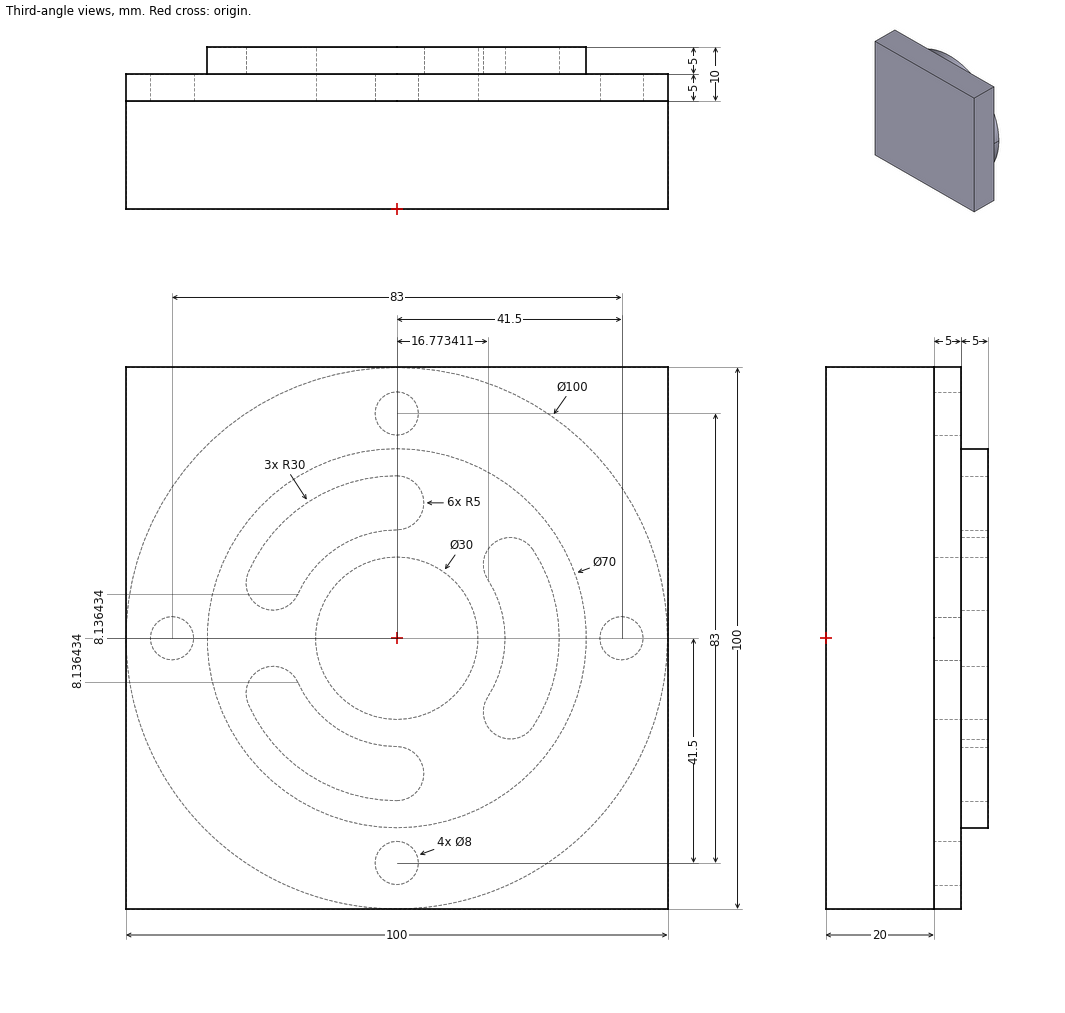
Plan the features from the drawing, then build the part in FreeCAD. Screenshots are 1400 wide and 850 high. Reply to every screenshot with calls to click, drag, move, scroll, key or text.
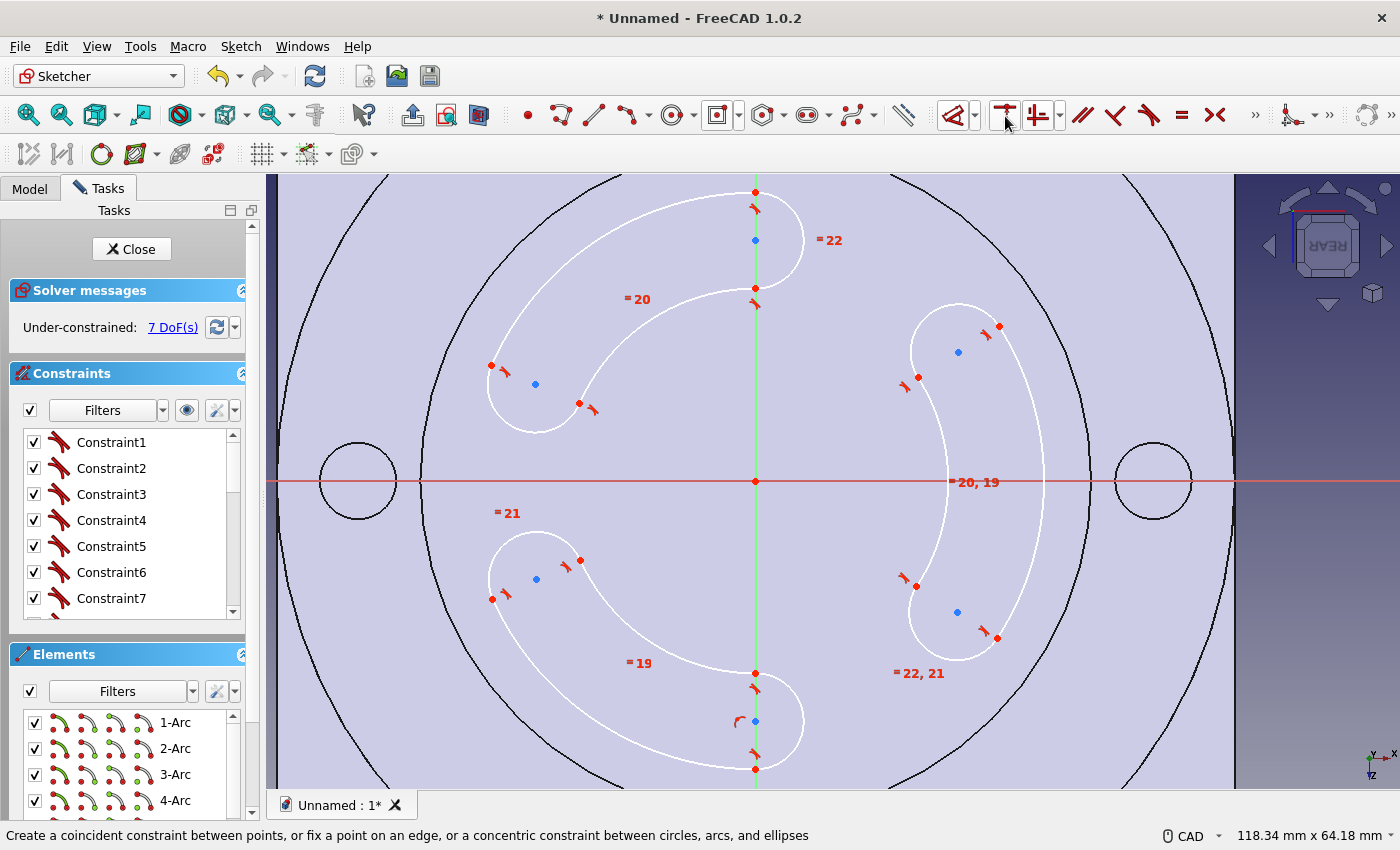
click(756, 241)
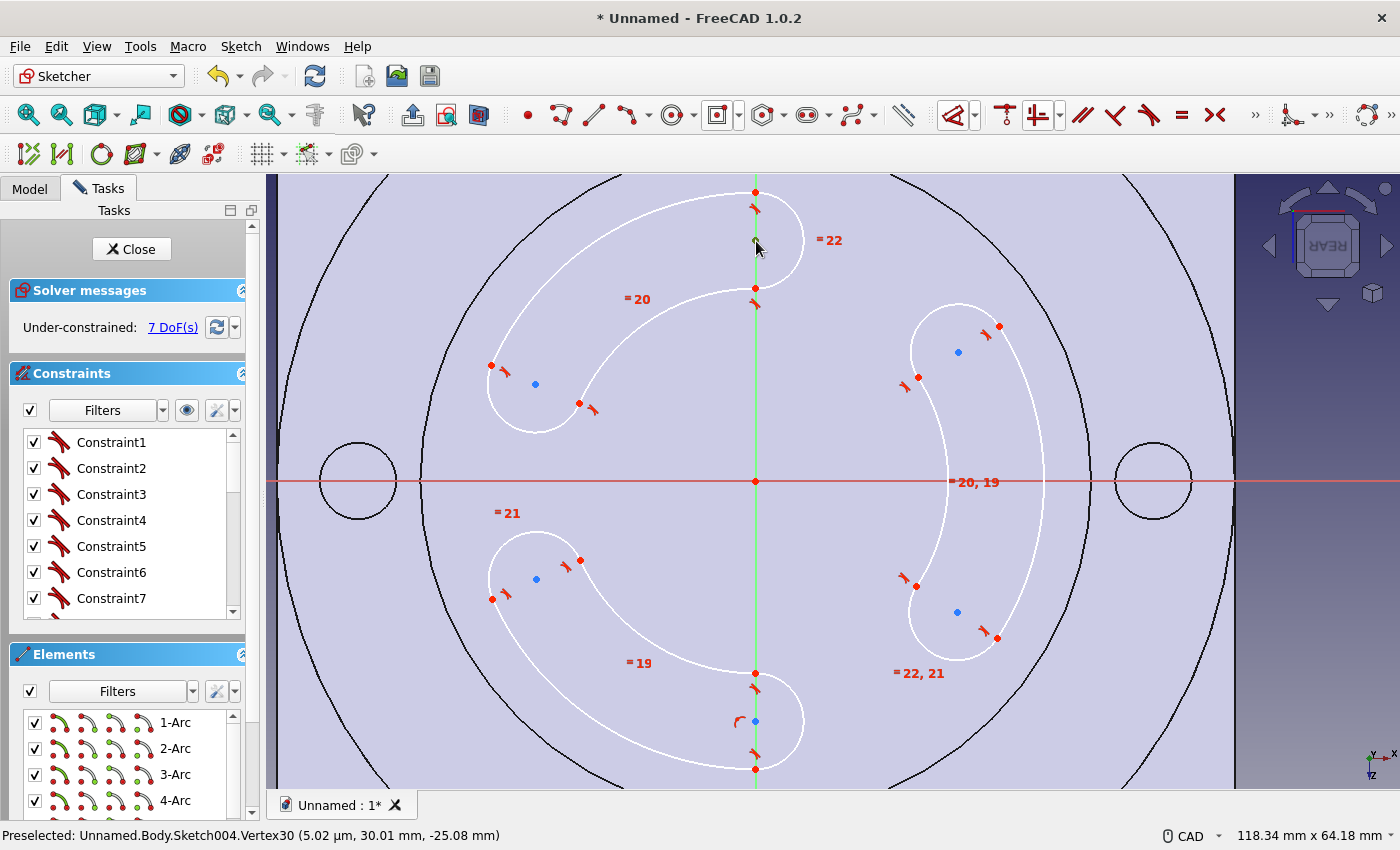
click(756, 641)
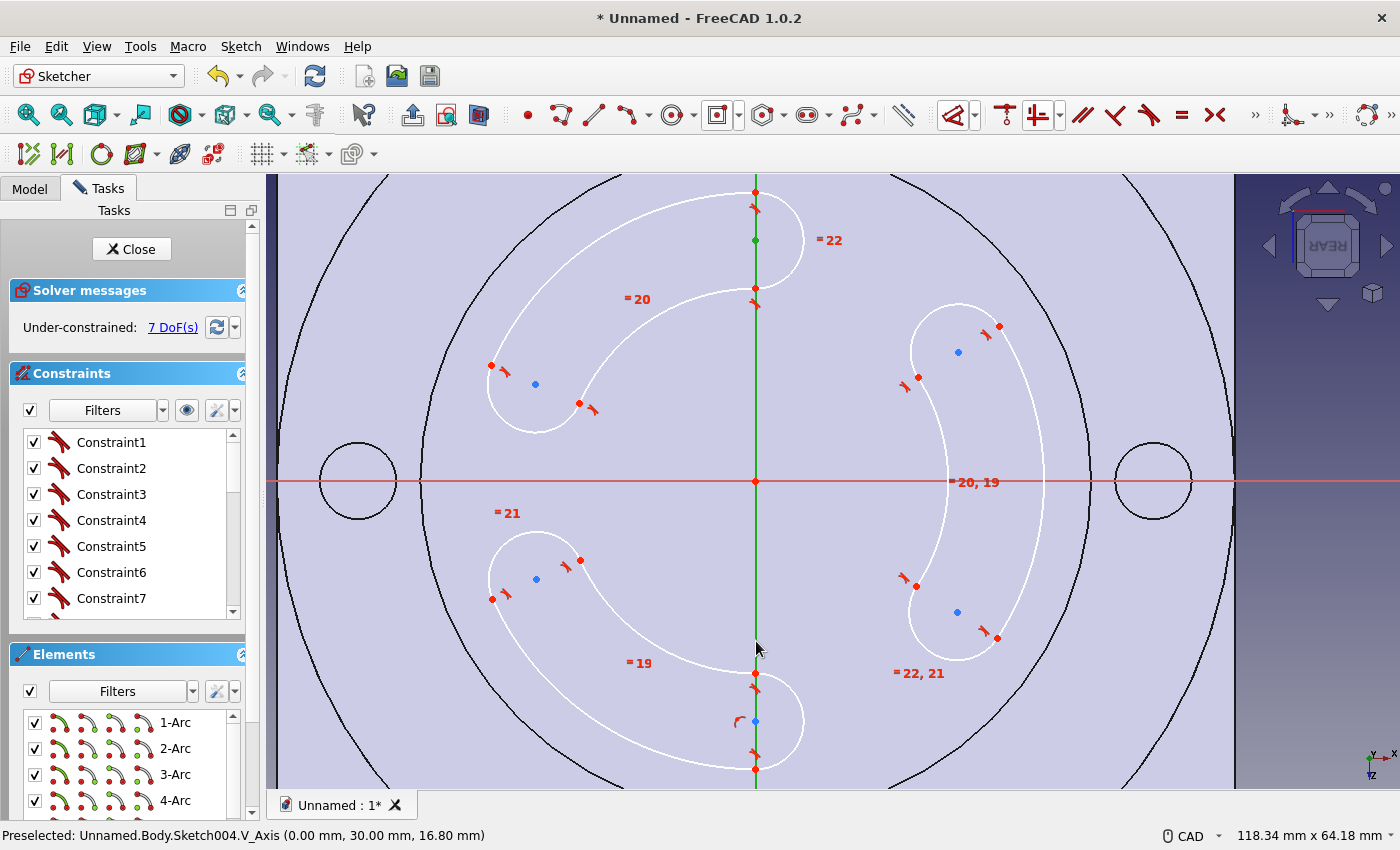
click(1005, 116)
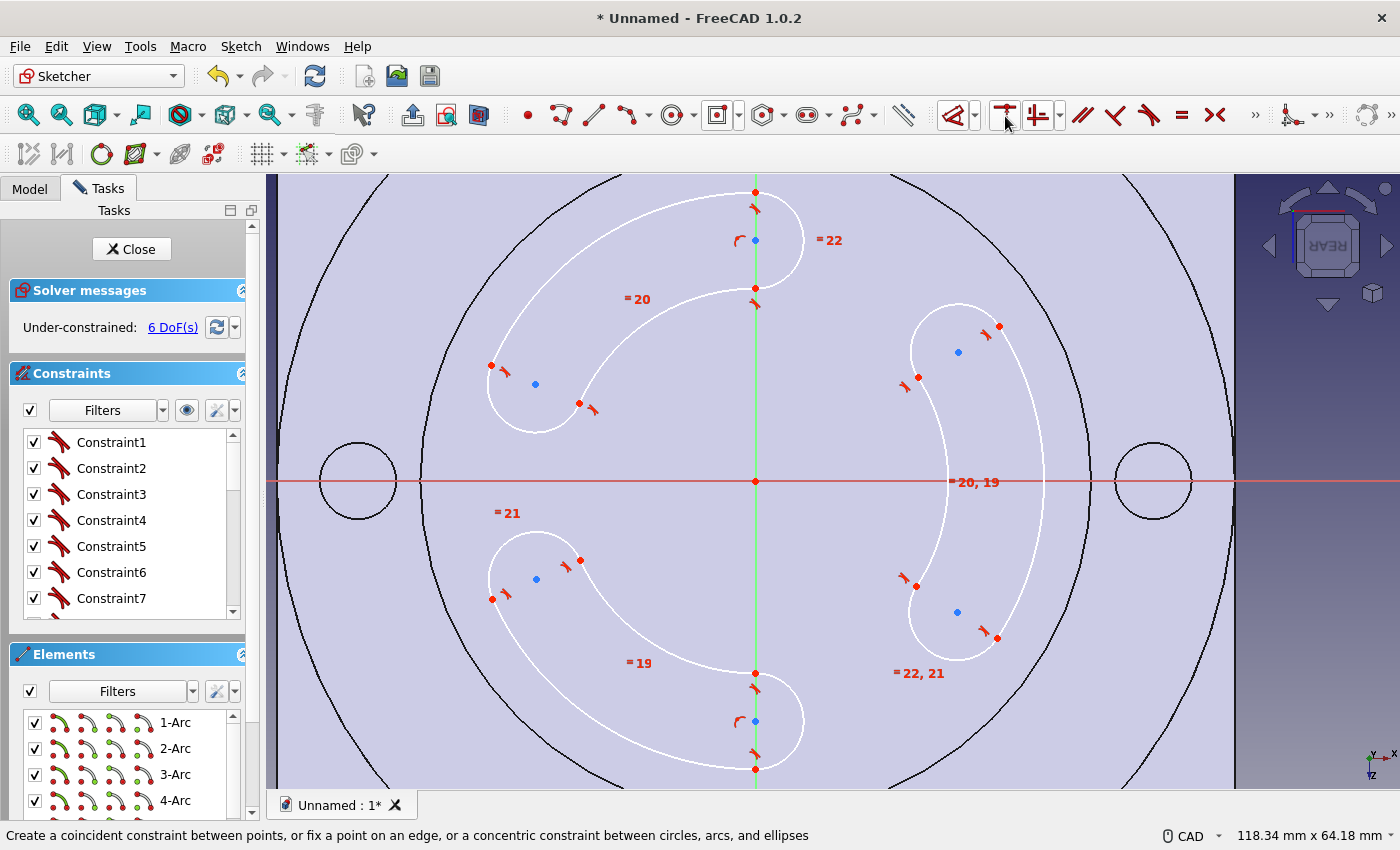
click(546, 533)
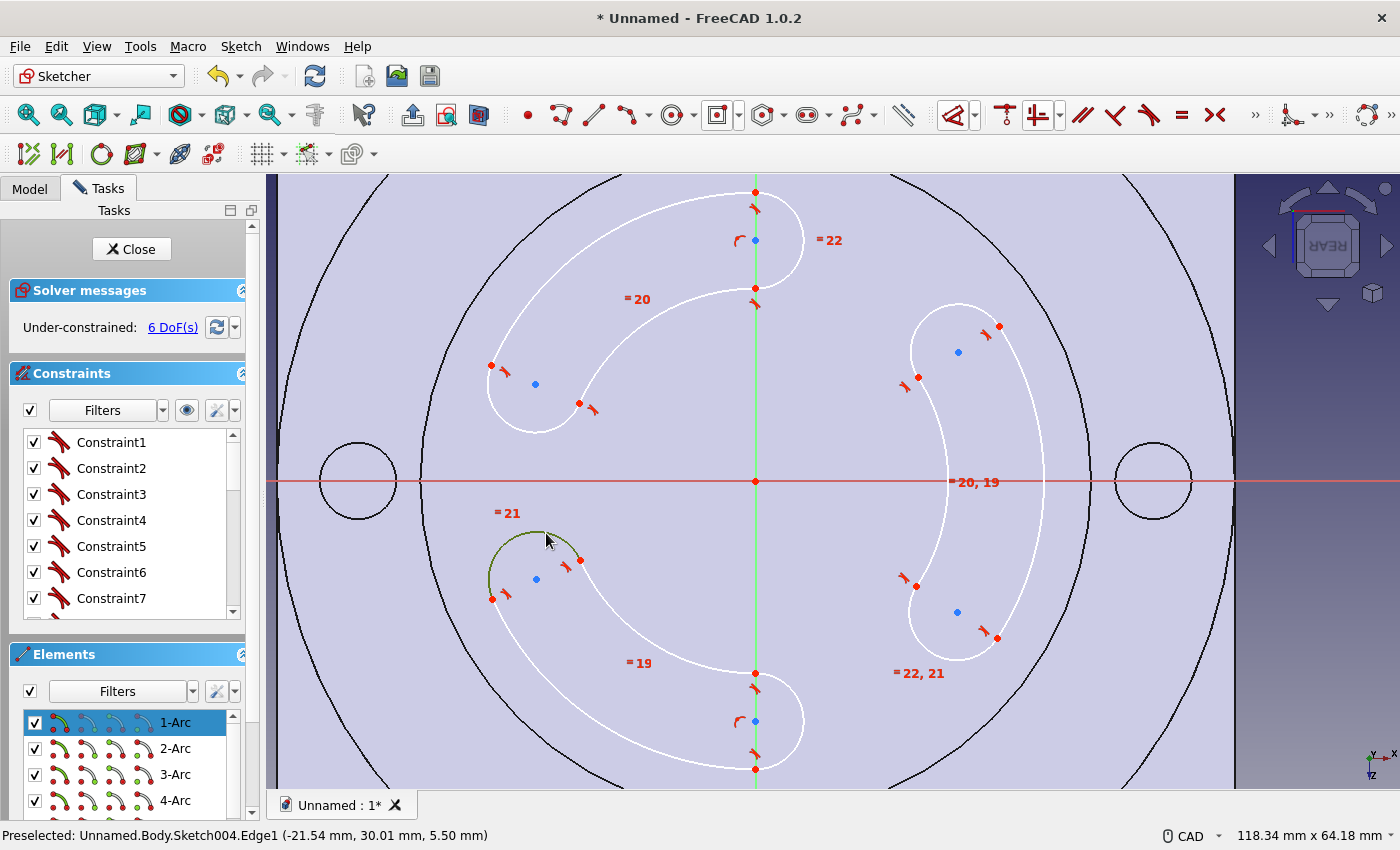
click(974, 116)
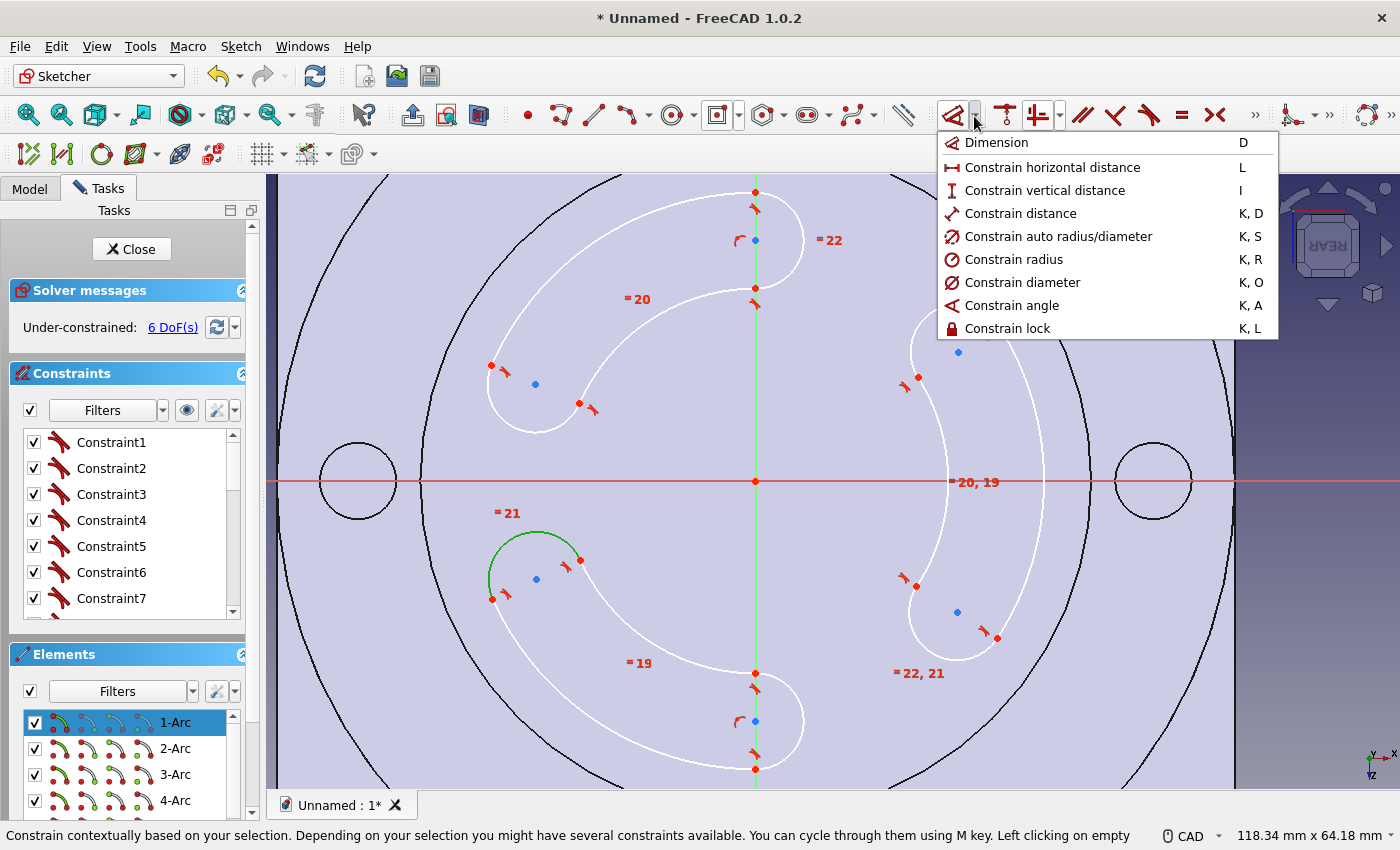
click(1108, 260)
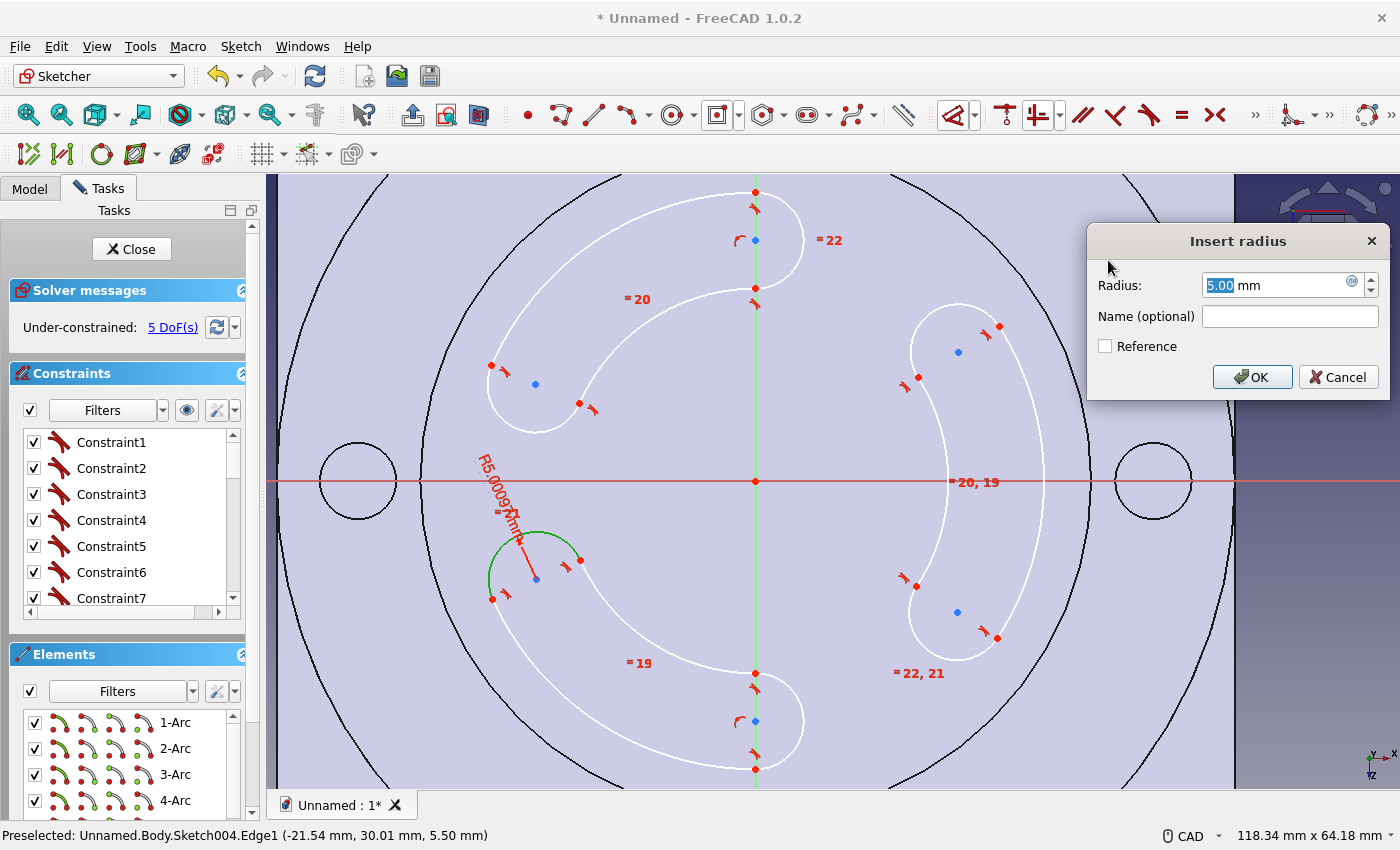
text(5)
key(Return)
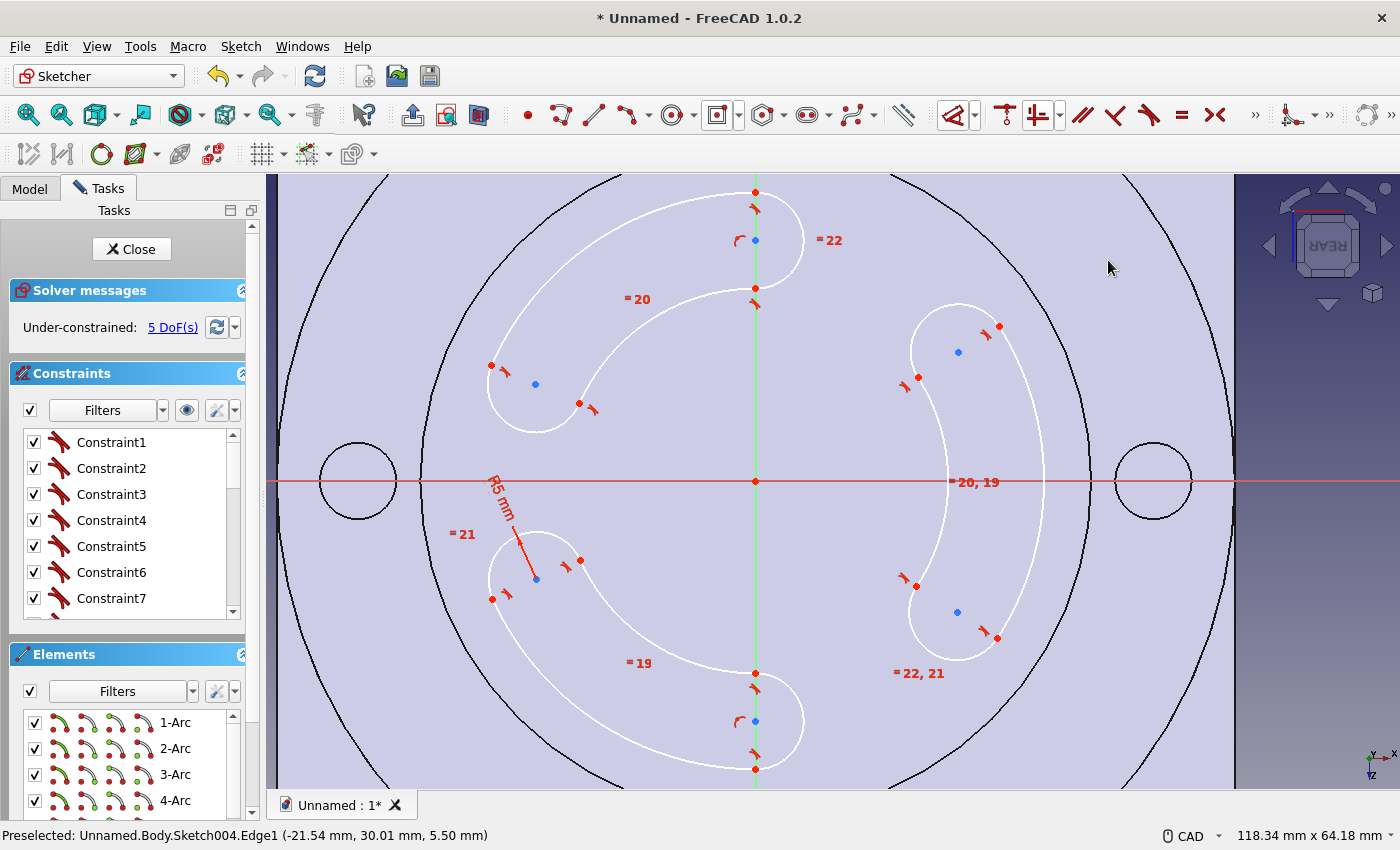
click(548, 681)